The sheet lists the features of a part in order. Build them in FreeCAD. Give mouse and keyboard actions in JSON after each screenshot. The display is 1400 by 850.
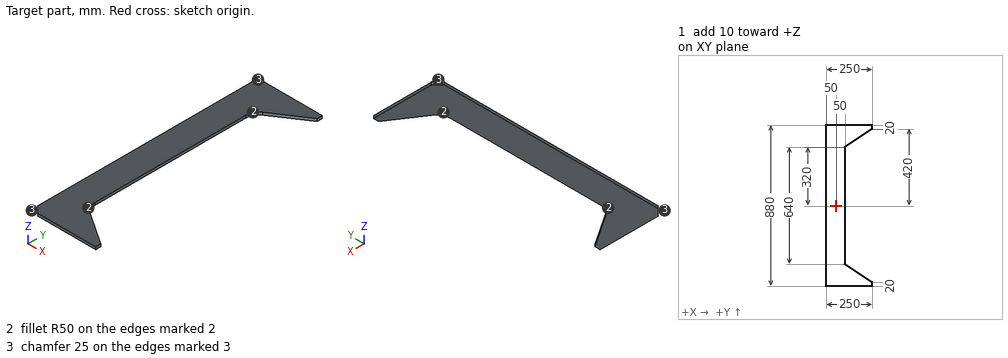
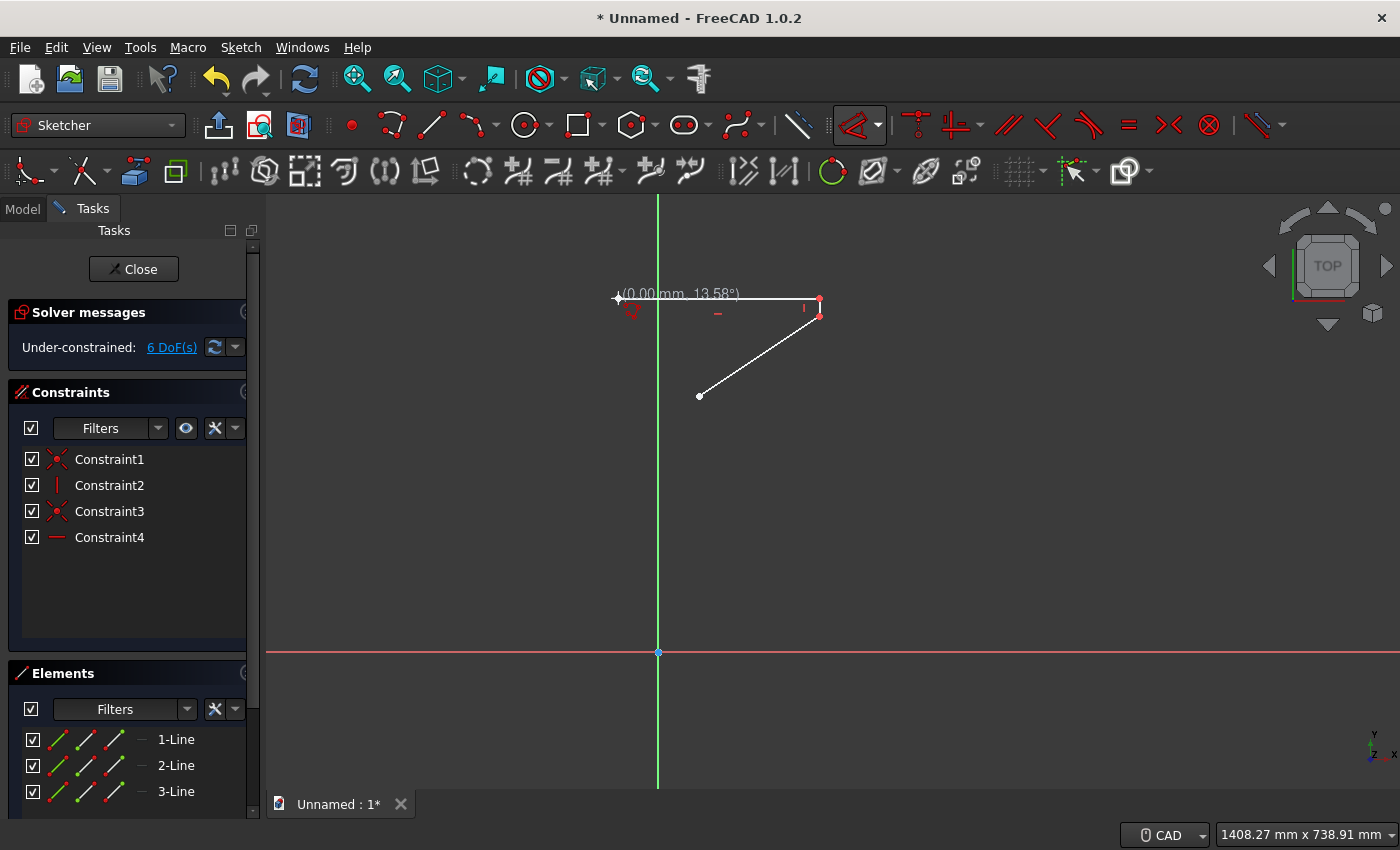
{"action": "scroll", "coordinate": [820, 296], "scroll_direction": "down", "scroll_amount": 3}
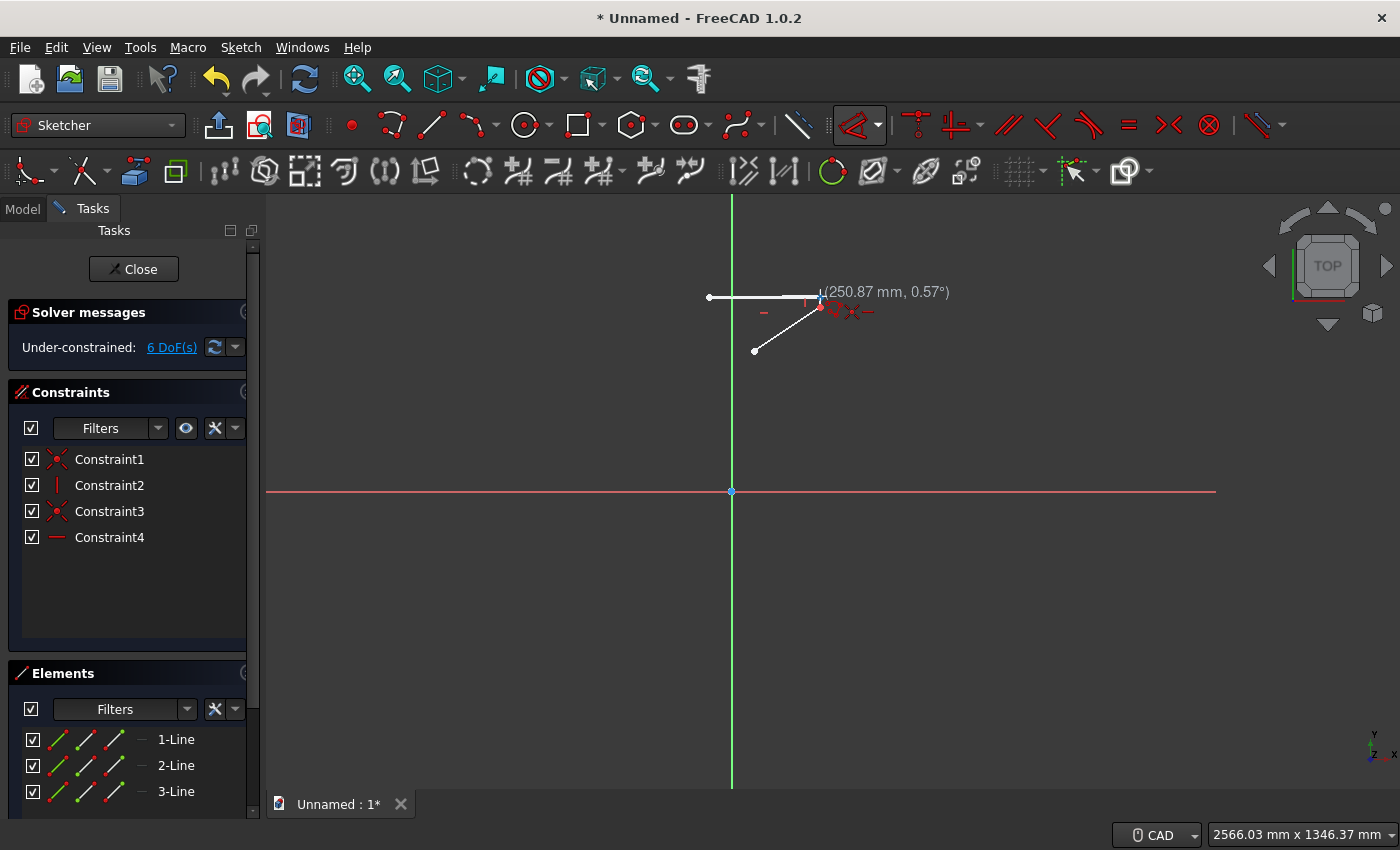
{"action": "left_click", "coordinate": [709, 686]}
{"action": "left_click", "coordinate": [820, 686]}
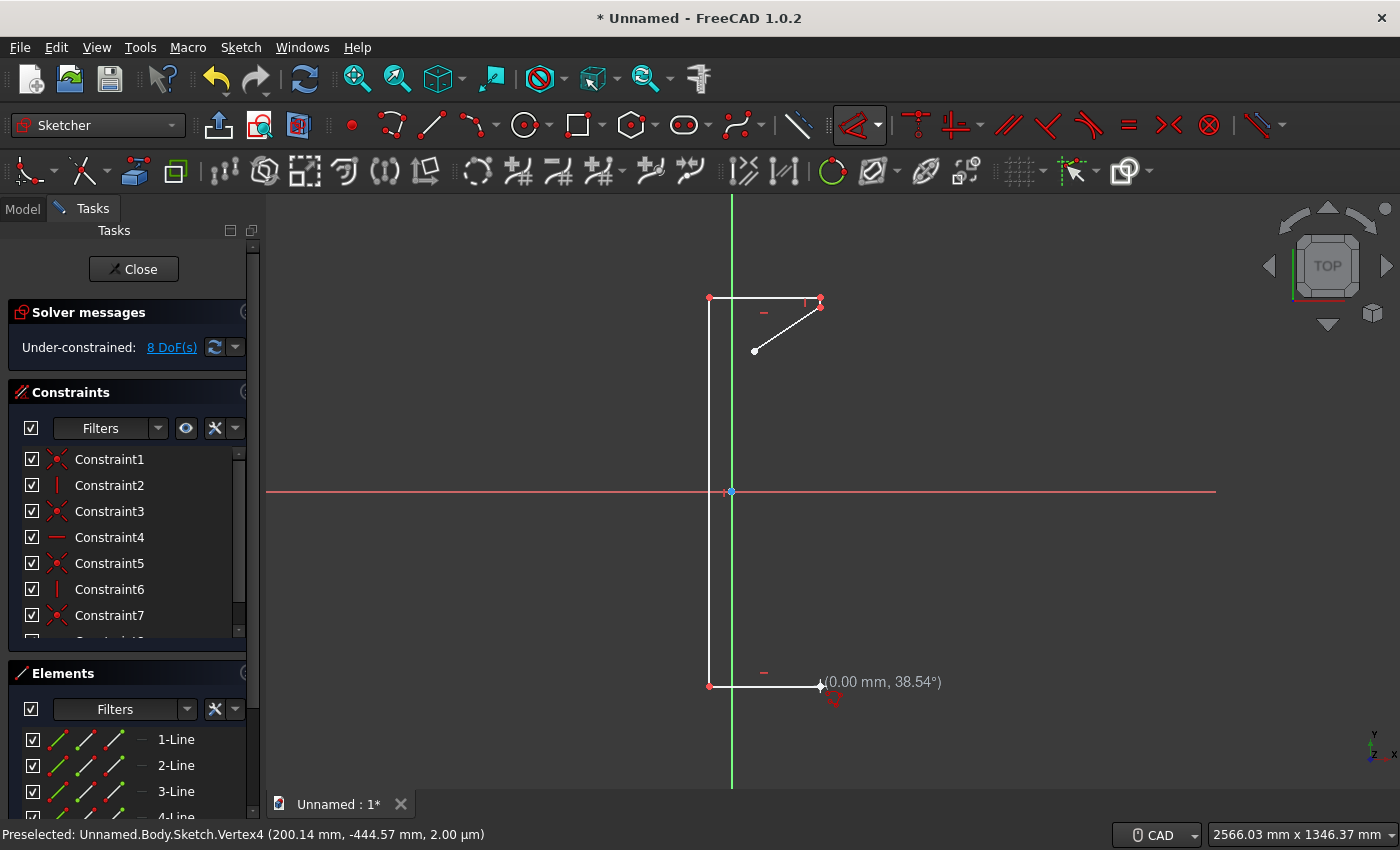
{"action": "scroll", "coordinate": [820, 677], "scroll_direction": "up", "scroll_amount": 3}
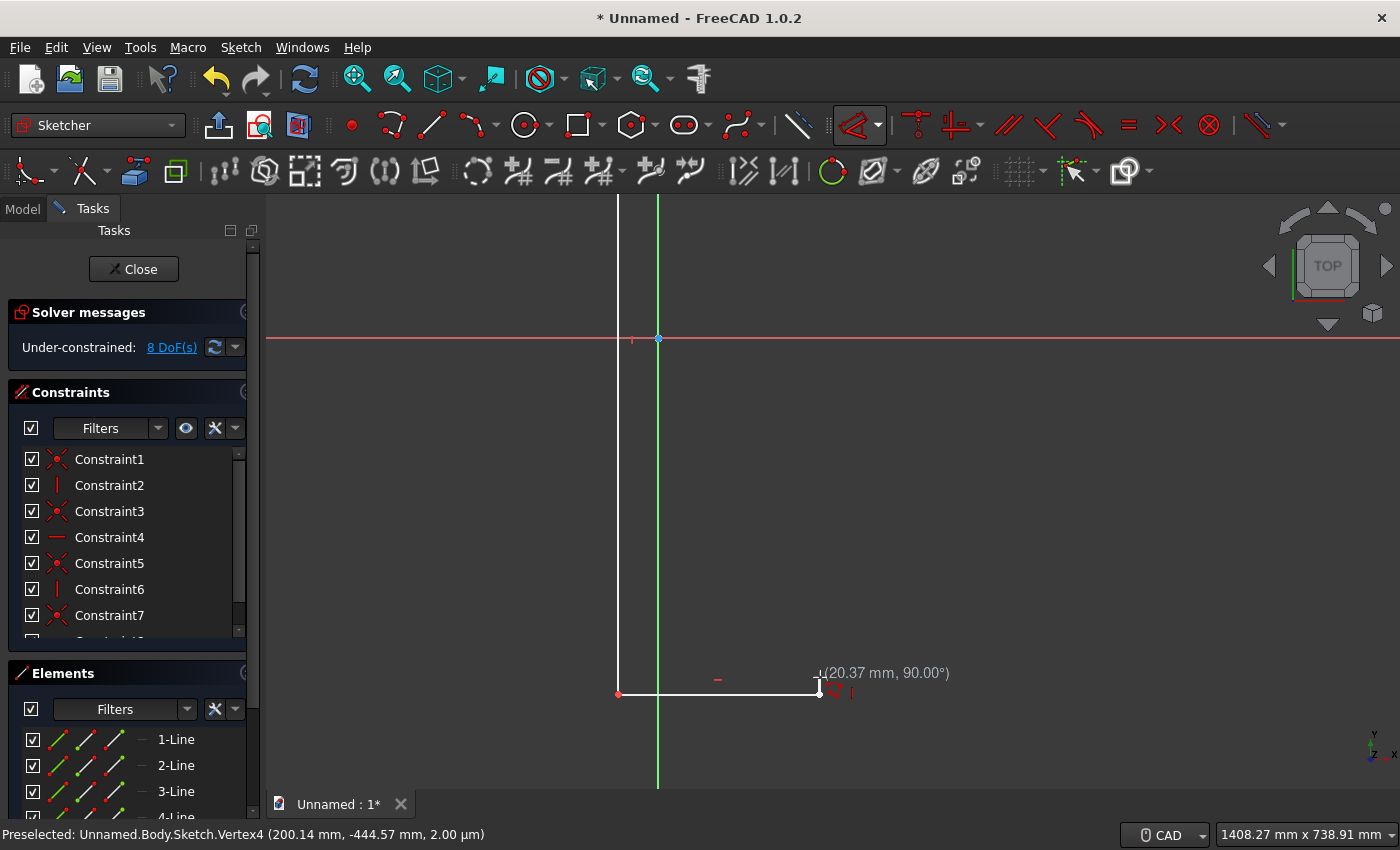
{"action": "left_click", "coordinate": [820, 677]}
{"action": "left_click", "coordinate": [699, 596]}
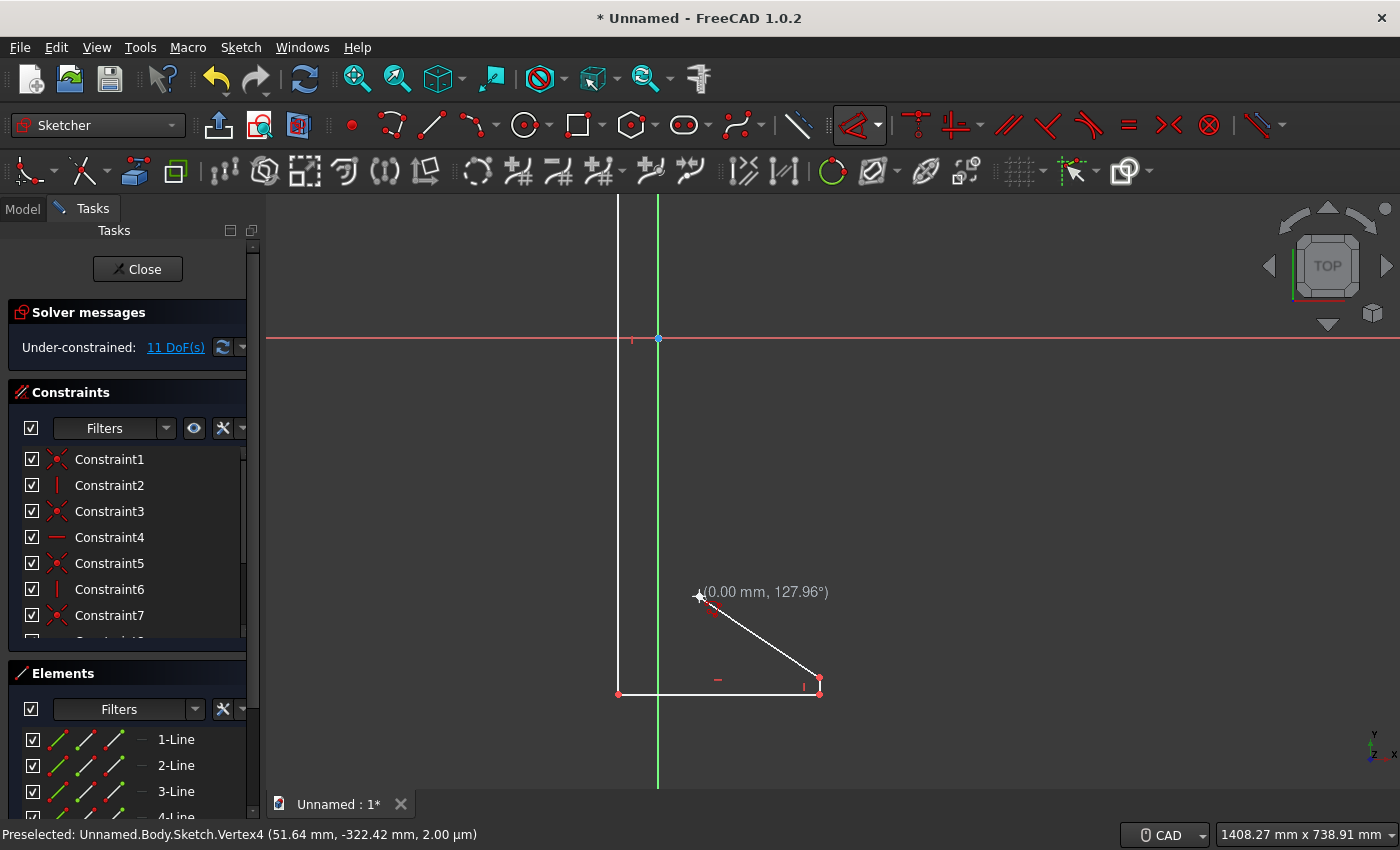
{"action": "scroll", "coordinate": [820, 678], "scroll_direction": "down", "scroll_amount": 3}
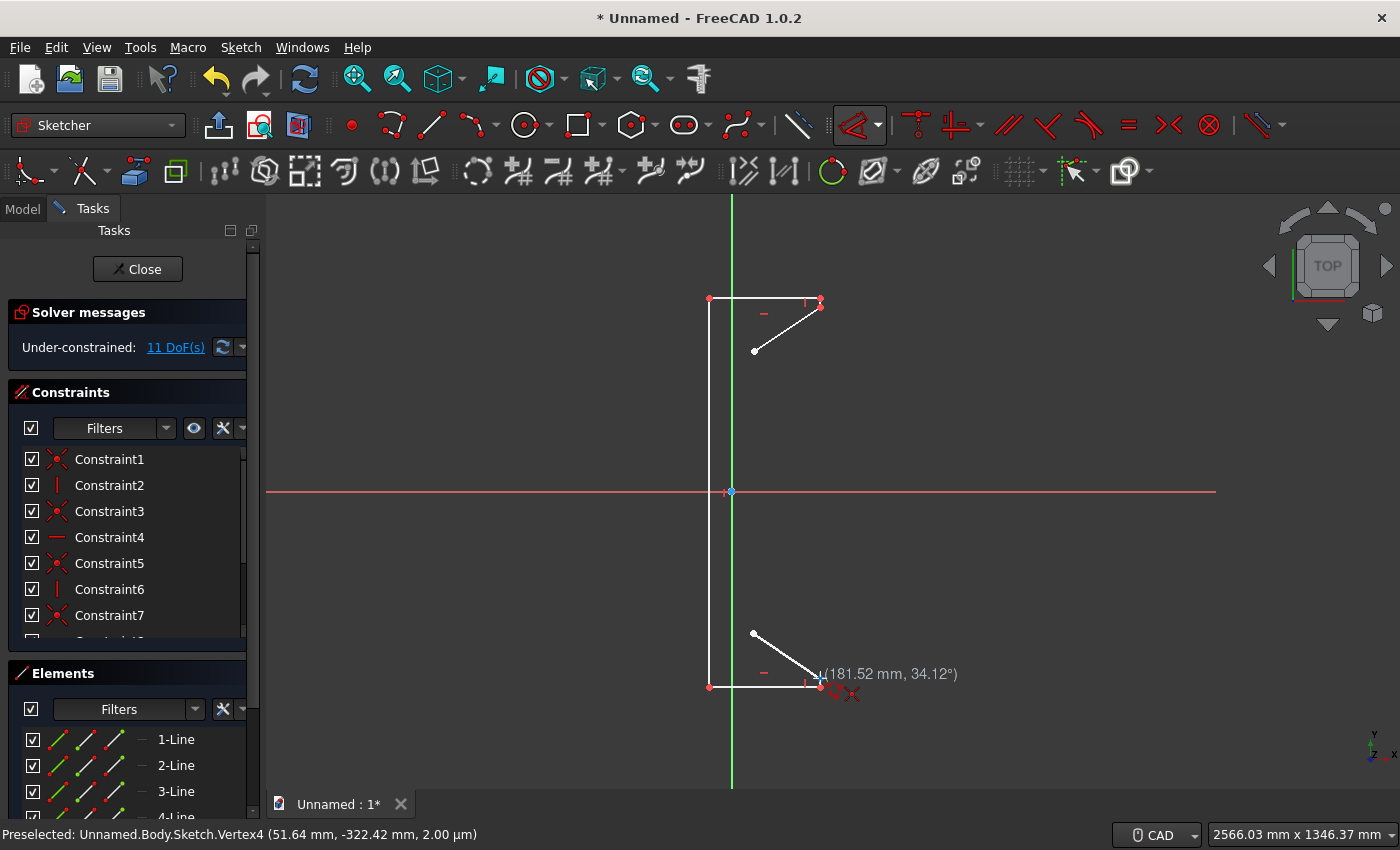
{"action": "left_click", "coordinate": [754, 352]}
{"action": "key", "text": "Escape"}
{"action": "key", "text": "Escape"}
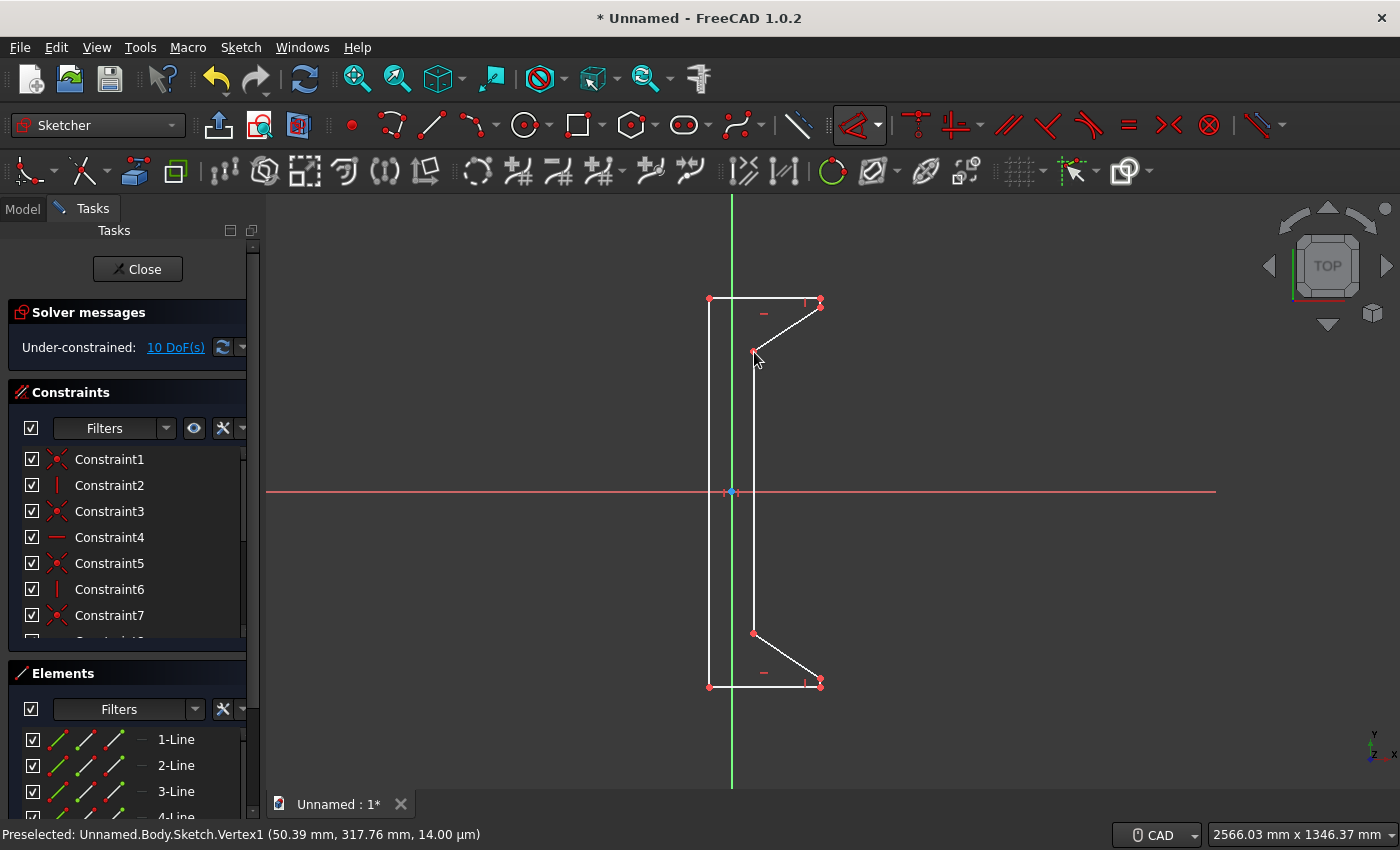
{"action": "left_click", "coordinate": [854, 126]}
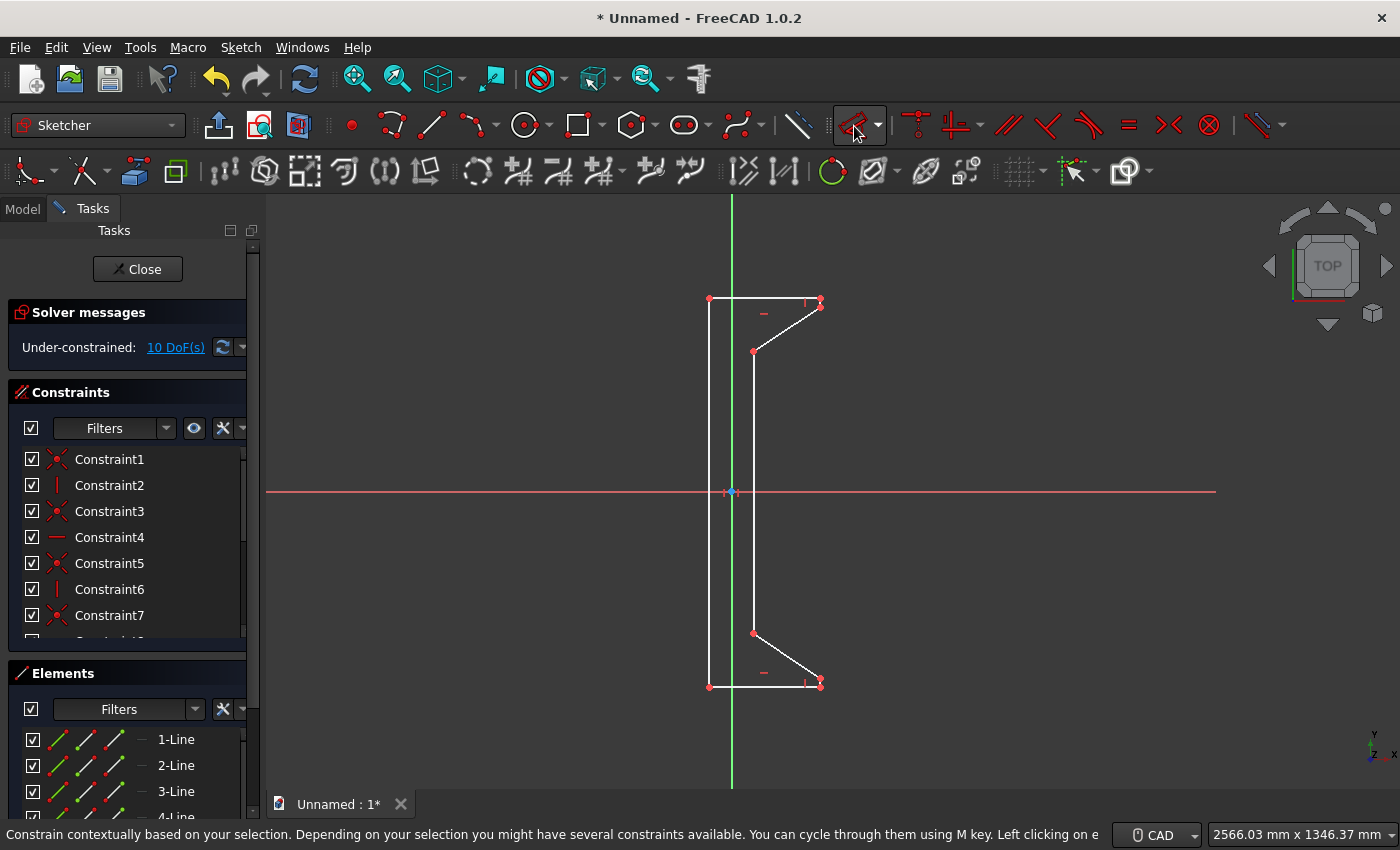
{"action": "scroll", "coordinate": [820, 303], "scroll_direction": "up", "scroll_amount": 8}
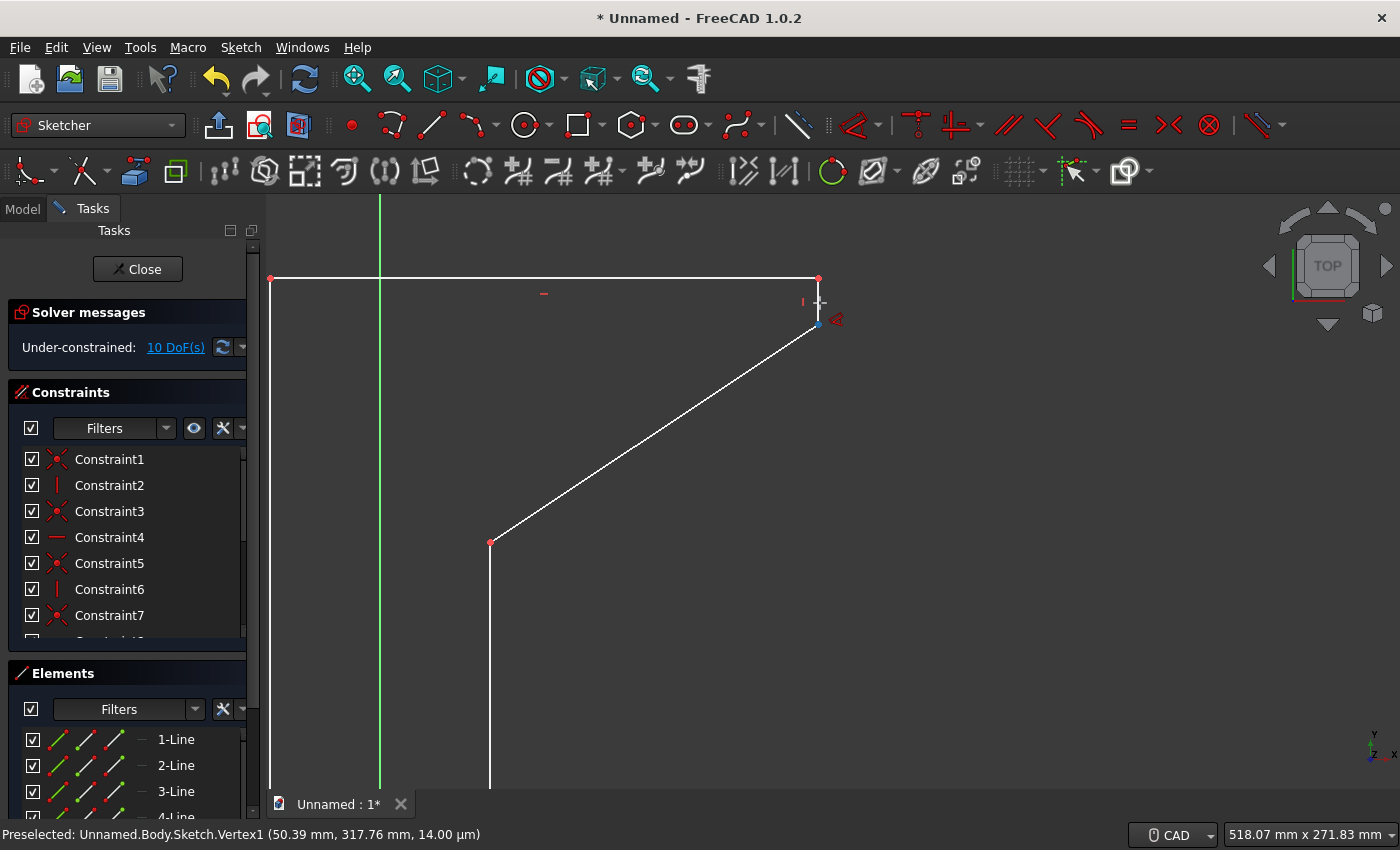
{"action": "left_click", "coordinate": [818, 302]}
{"action": "left_click", "coordinate": [852, 302]}